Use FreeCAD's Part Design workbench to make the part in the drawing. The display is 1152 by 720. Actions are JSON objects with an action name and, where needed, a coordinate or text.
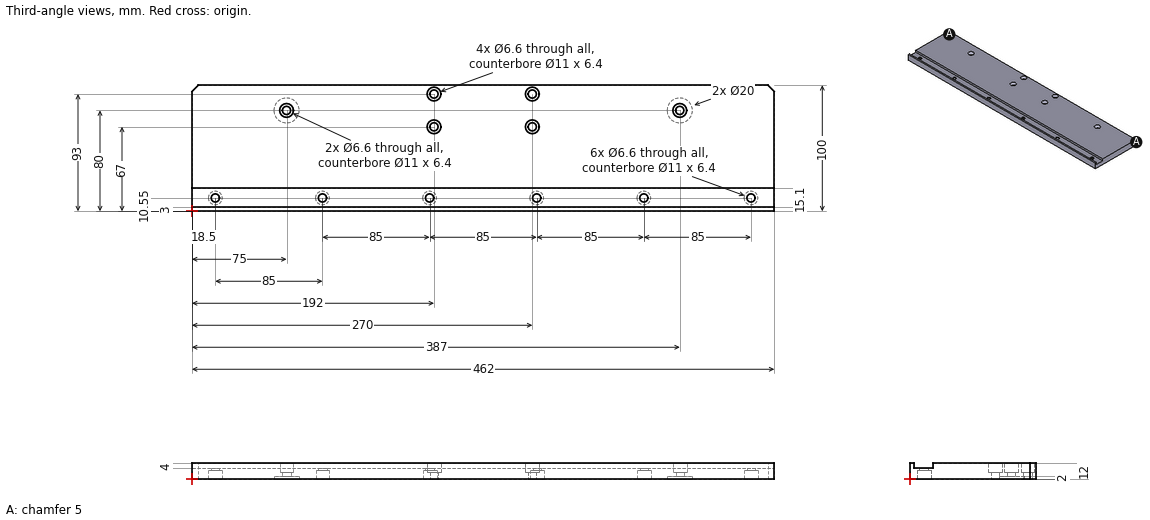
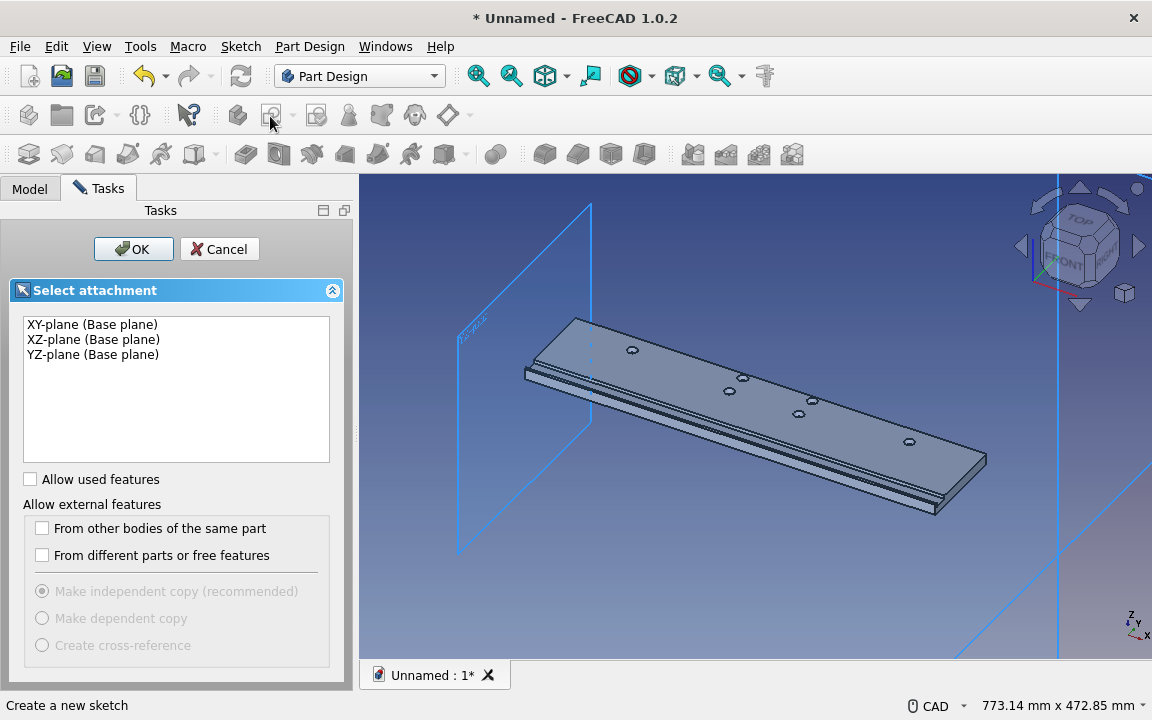
{"action": "left_click", "coordinate": [84, 324]}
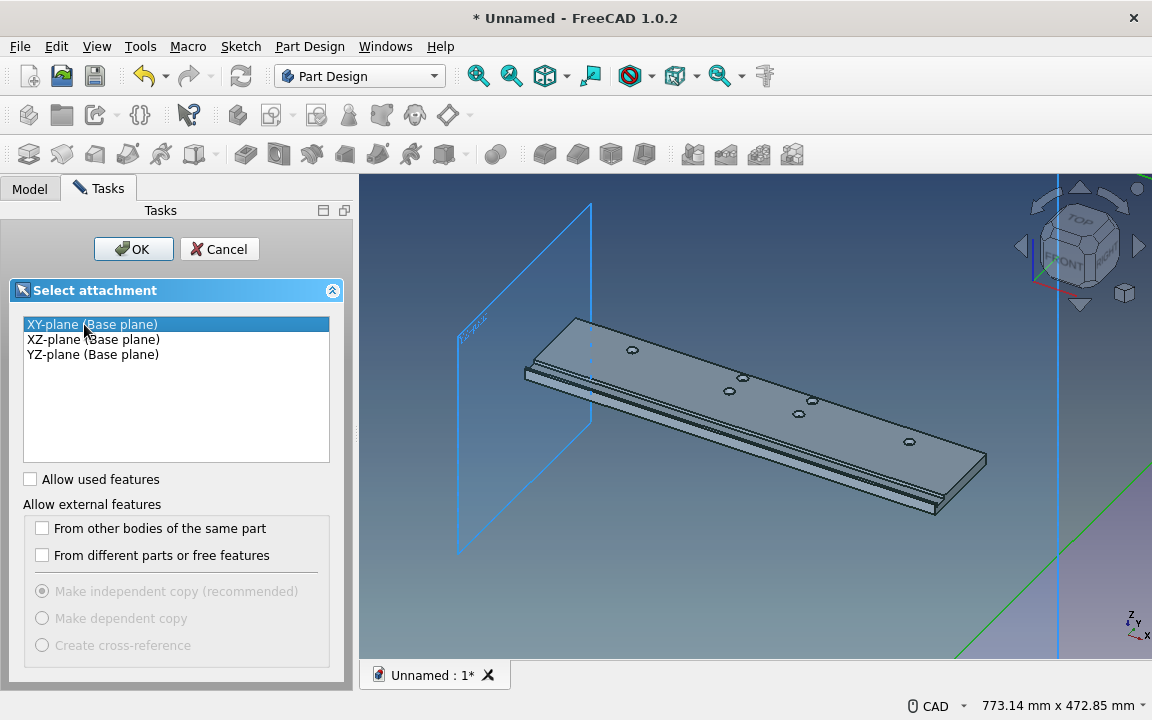
{"action": "left_click", "coordinate": [134, 249]}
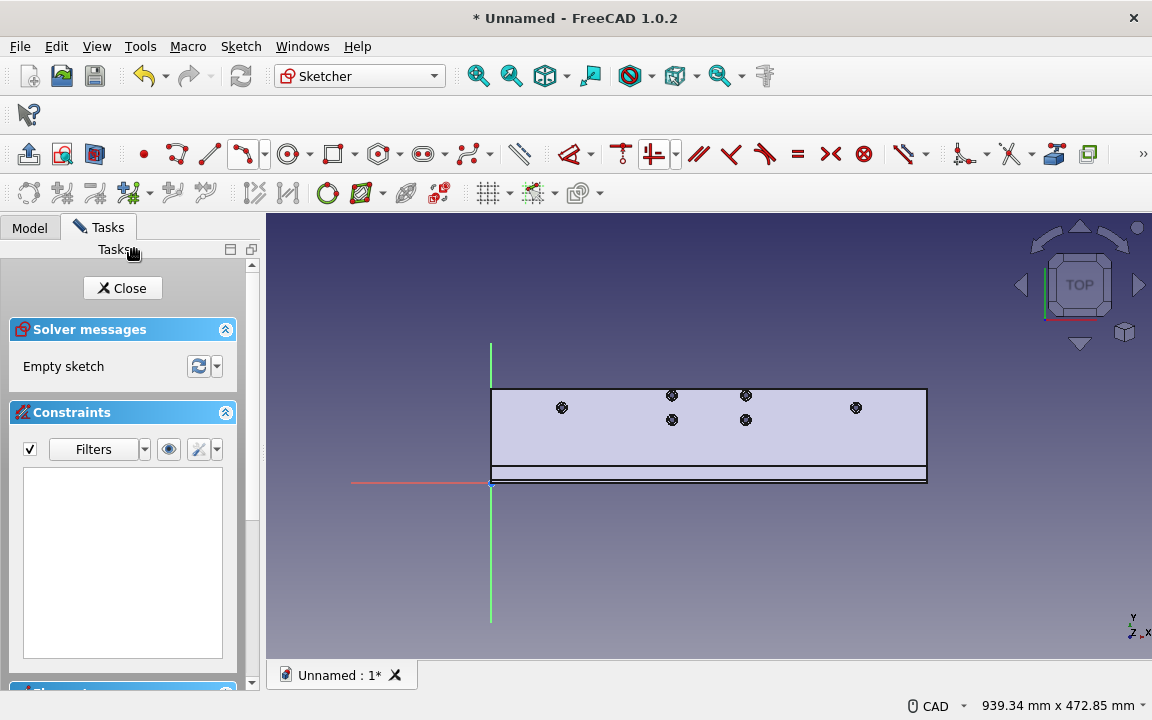
{"action": "key", "text": "q s"}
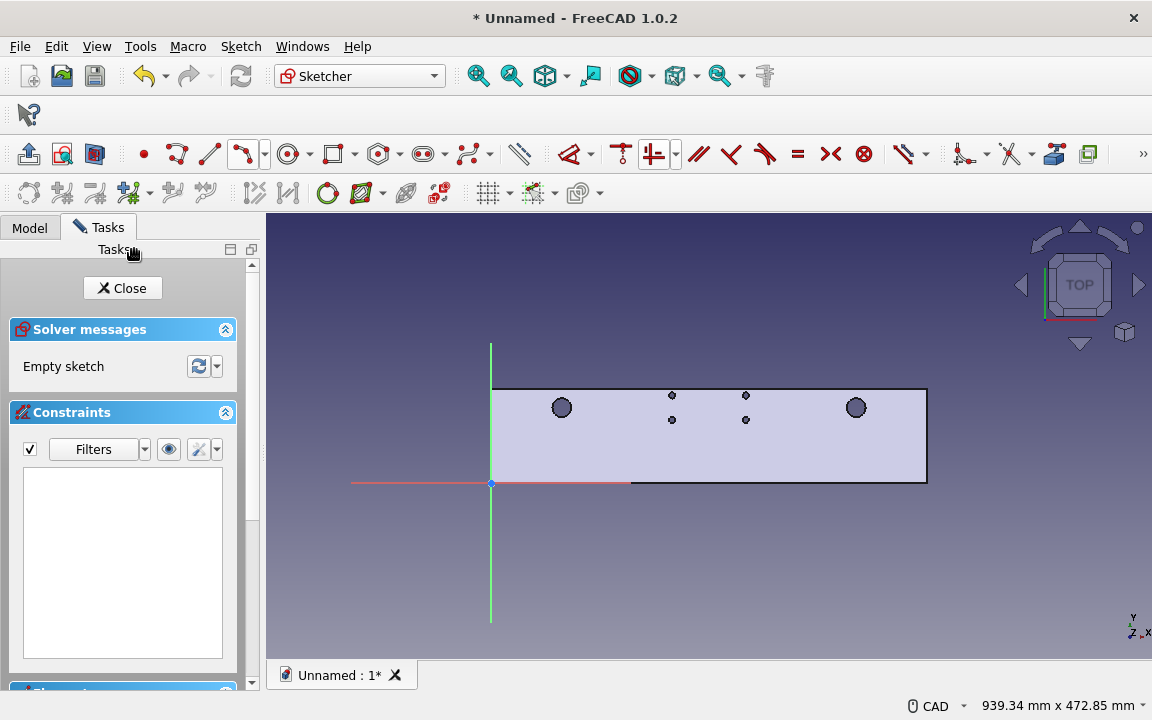
{"action": "left_click", "coordinate": [288, 154]}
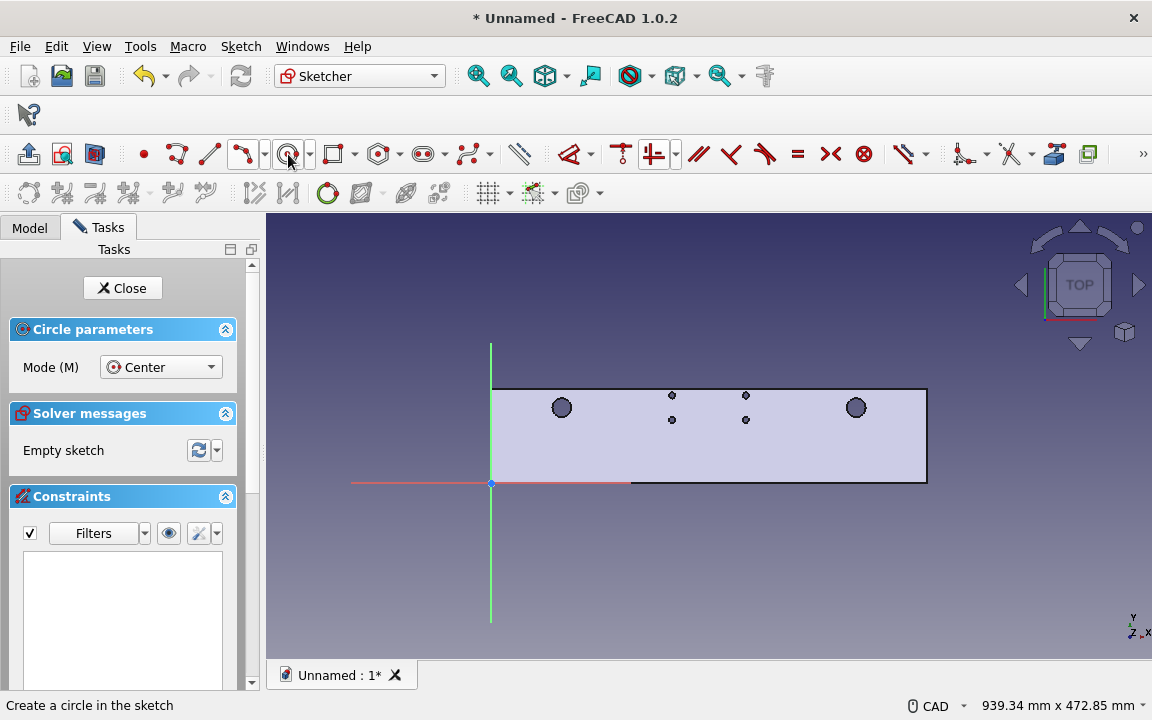
{"action": "scroll", "coordinate": [909, 473], "scroll_direction": "up", "scroll_amount": 10}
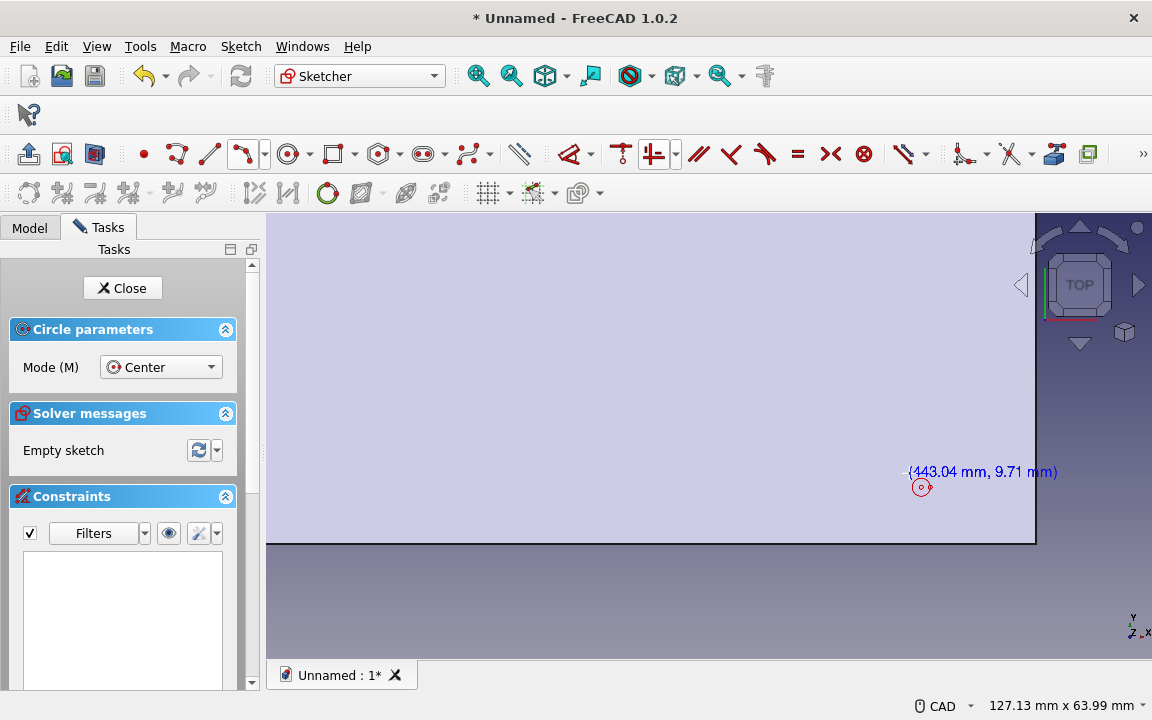
{"action": "scroll", "coordinate": [891, 424], "scroll_direction": "down", "scroll_amount": 9}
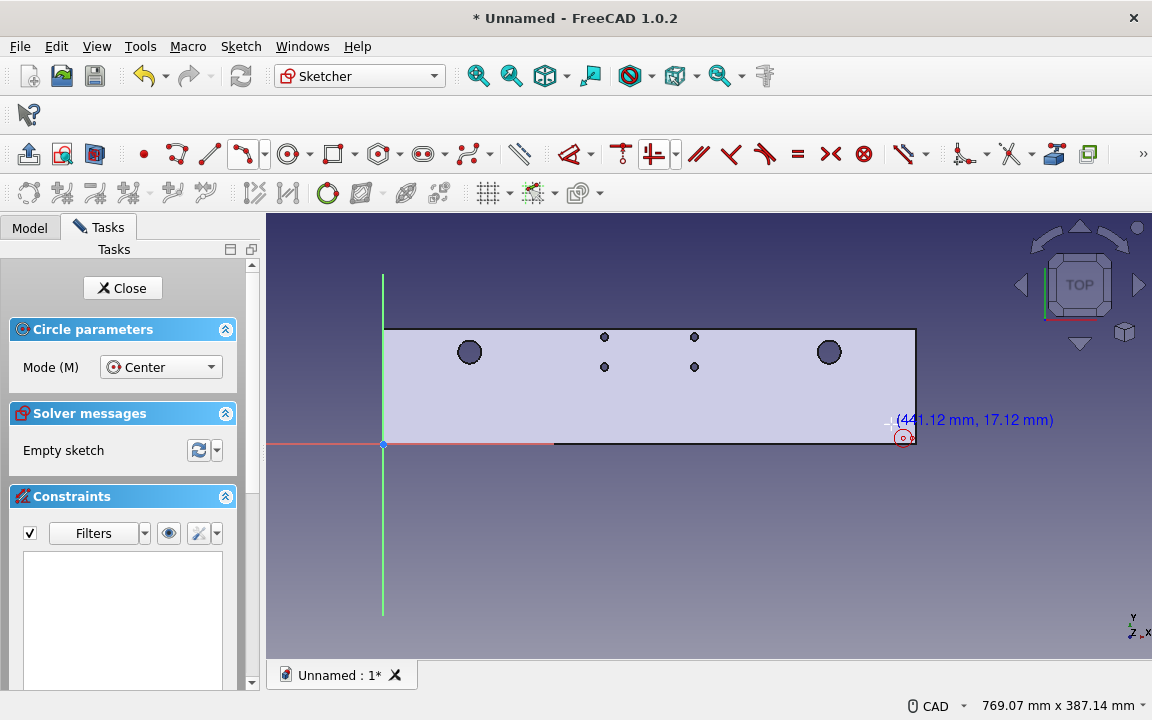
{"action": "scroll", "coordinate": [894, 432], "scroll_direction": "up", "scroll_amount": 2}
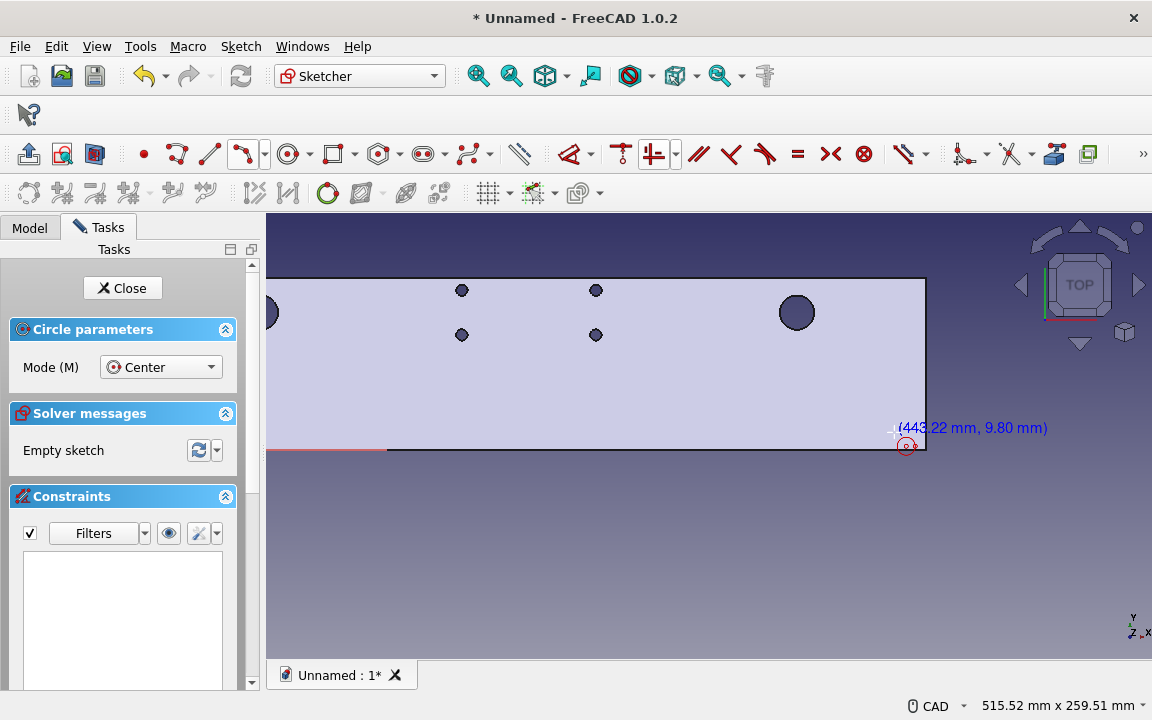
{"action": "left_click", "coordinate": [894, 432]}
{"action": "mouse_move", "coordinate": [898, 428]}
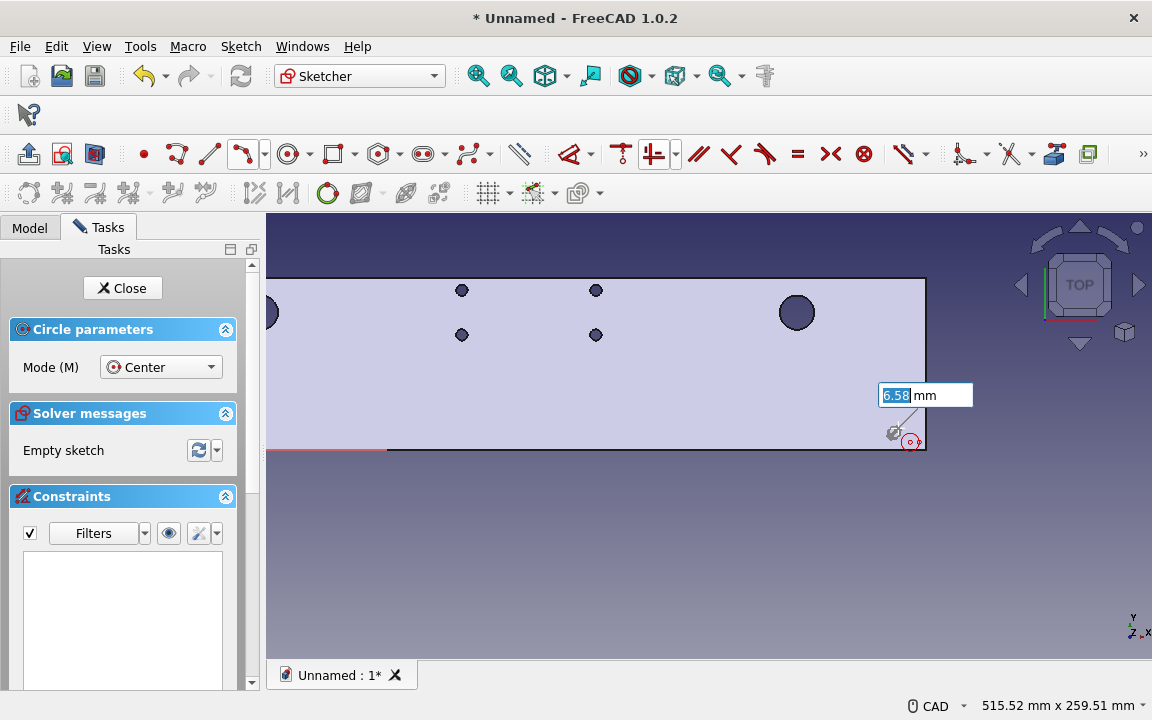
{"action": "type", "text": "6.6"}
{"action": "key", "text": "Return"}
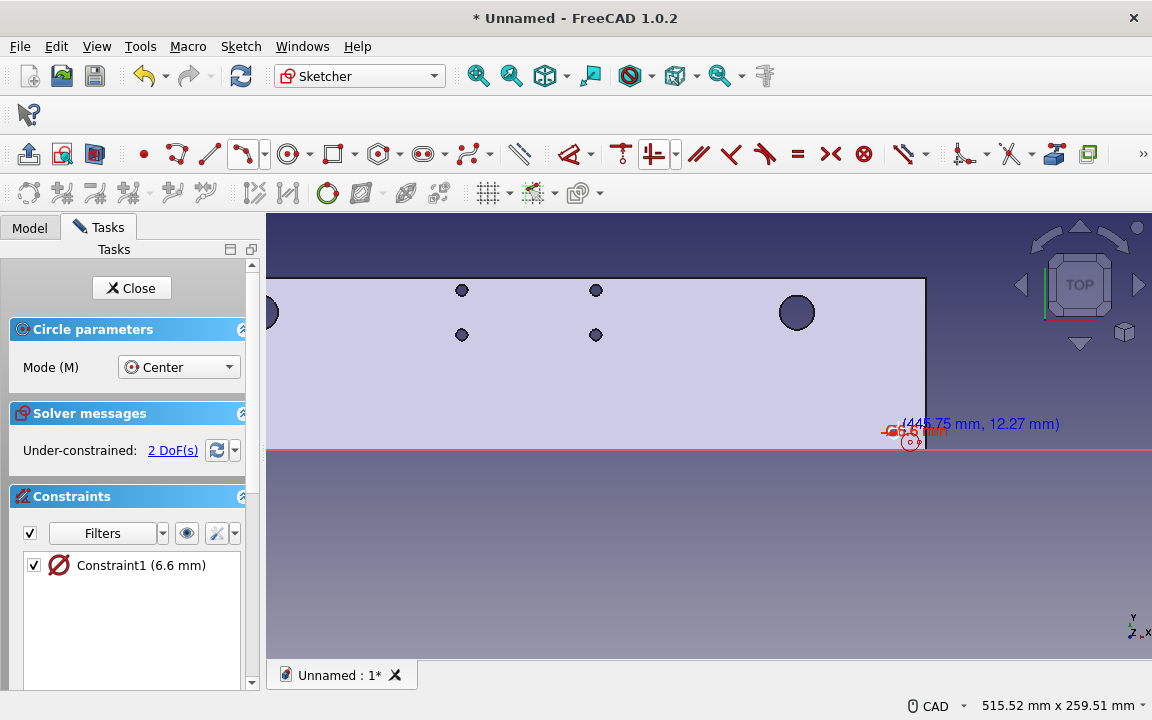
{"action": "scroll", "coordinate": [748, 432], "scroll_direction": "up", "scroll_amount": 7}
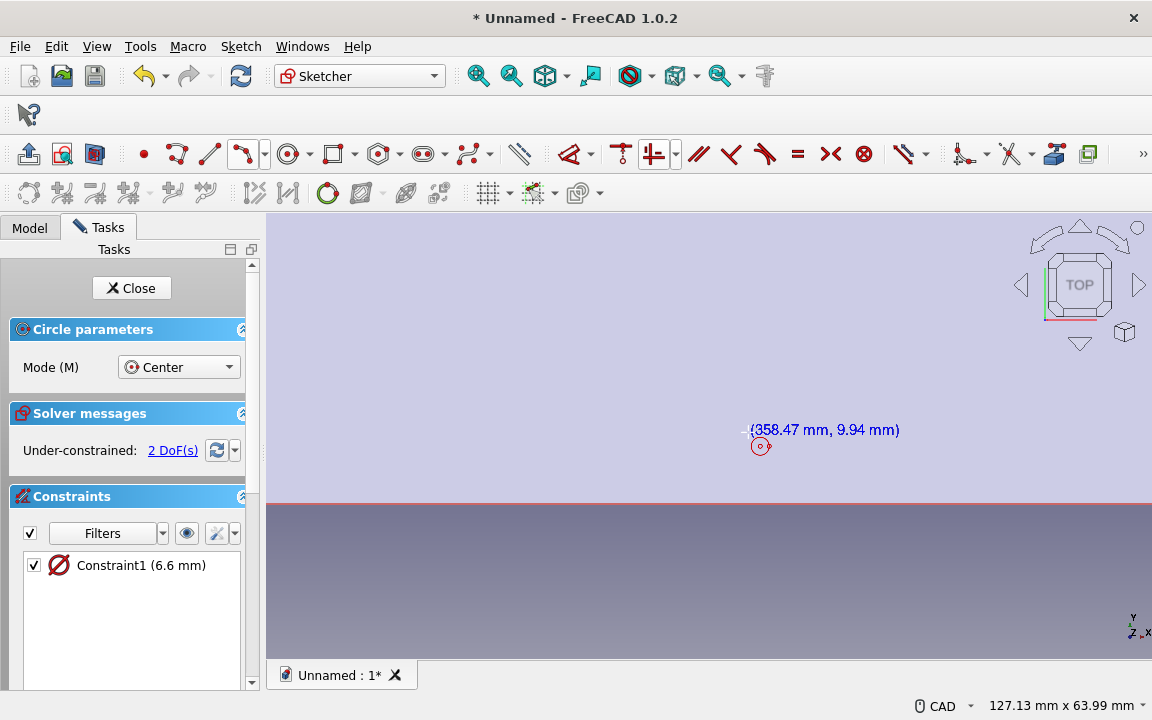
{"action": "scroll", "coordinate": [806, 432], "scroll_direction": "down", "scroll_amount": 9}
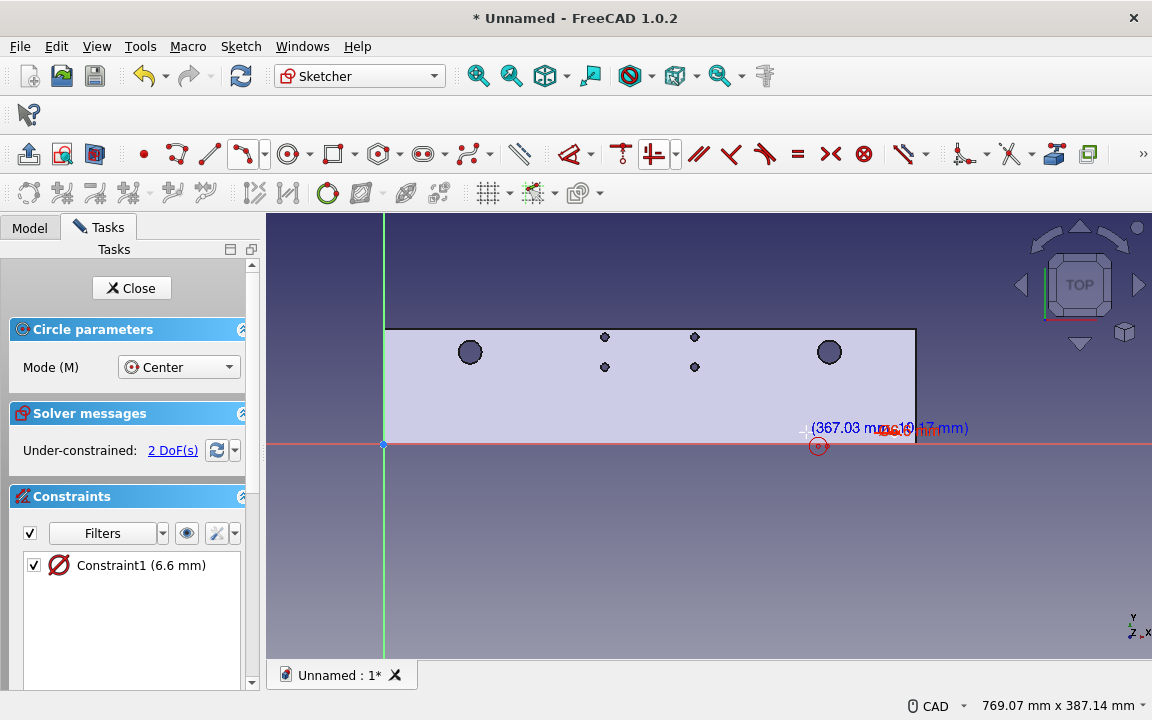
{"action": "scroll", "coordinate": [797, 432], "scroll_direction": "up", "scroll_amount": 2}